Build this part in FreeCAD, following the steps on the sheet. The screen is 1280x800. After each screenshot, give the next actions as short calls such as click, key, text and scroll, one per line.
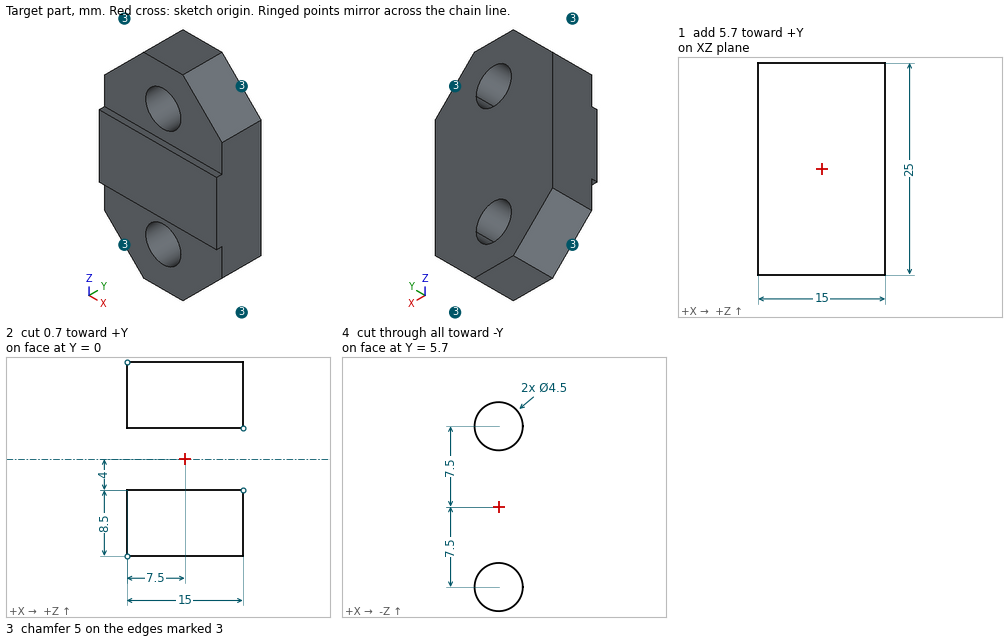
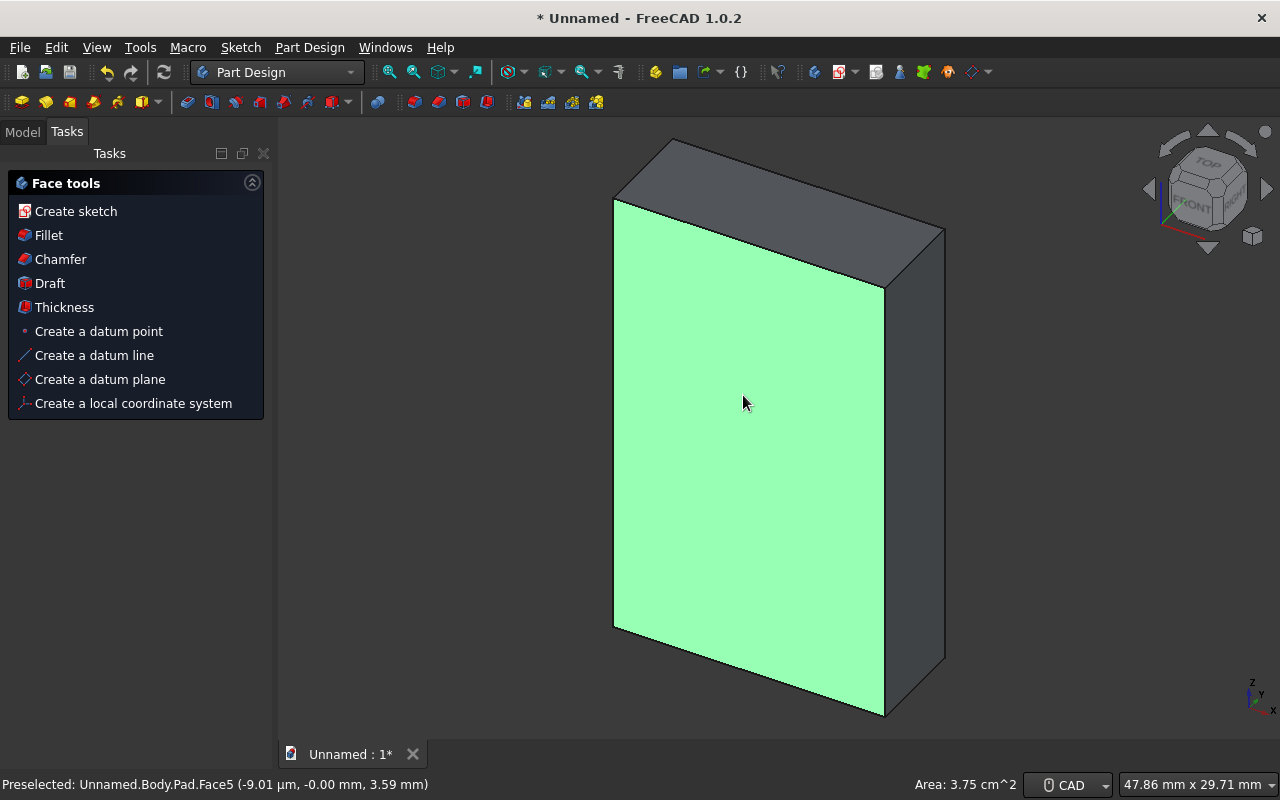
click(840, 72)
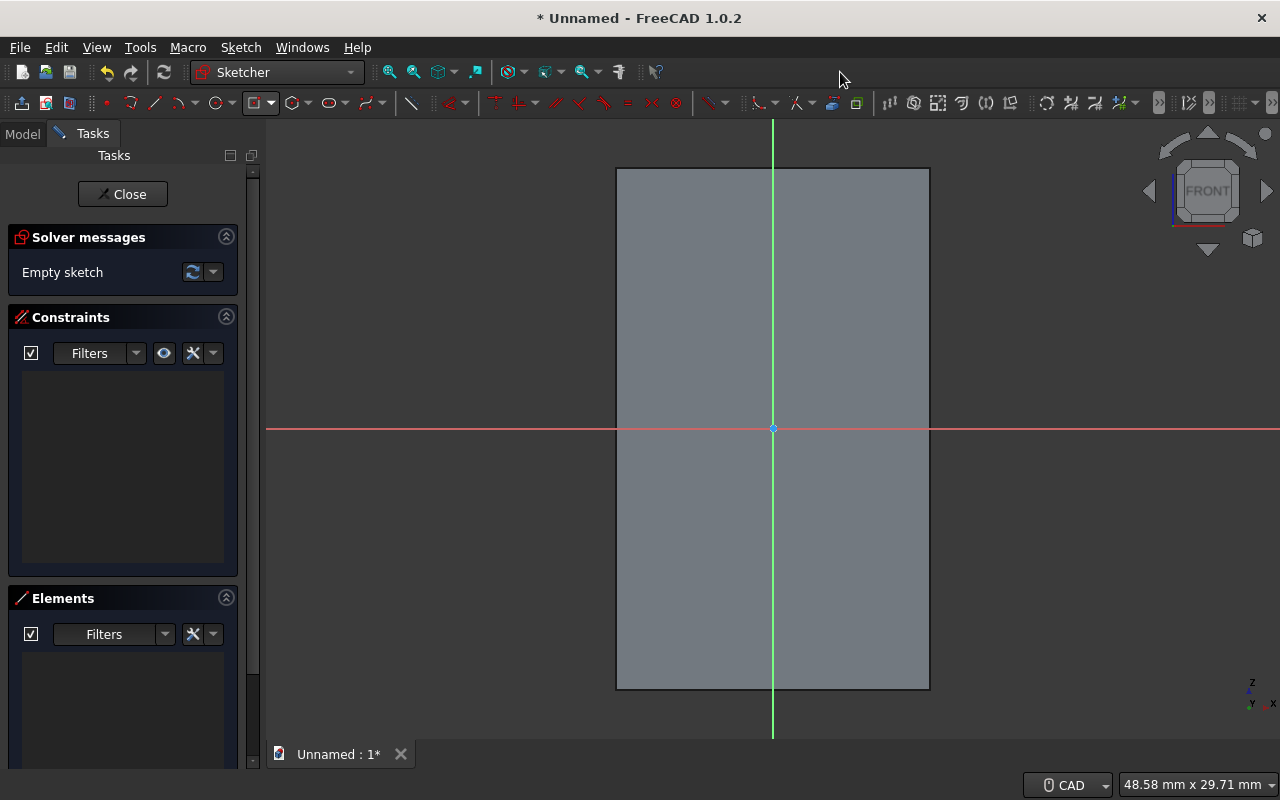
scroll(395, 429, down, 1)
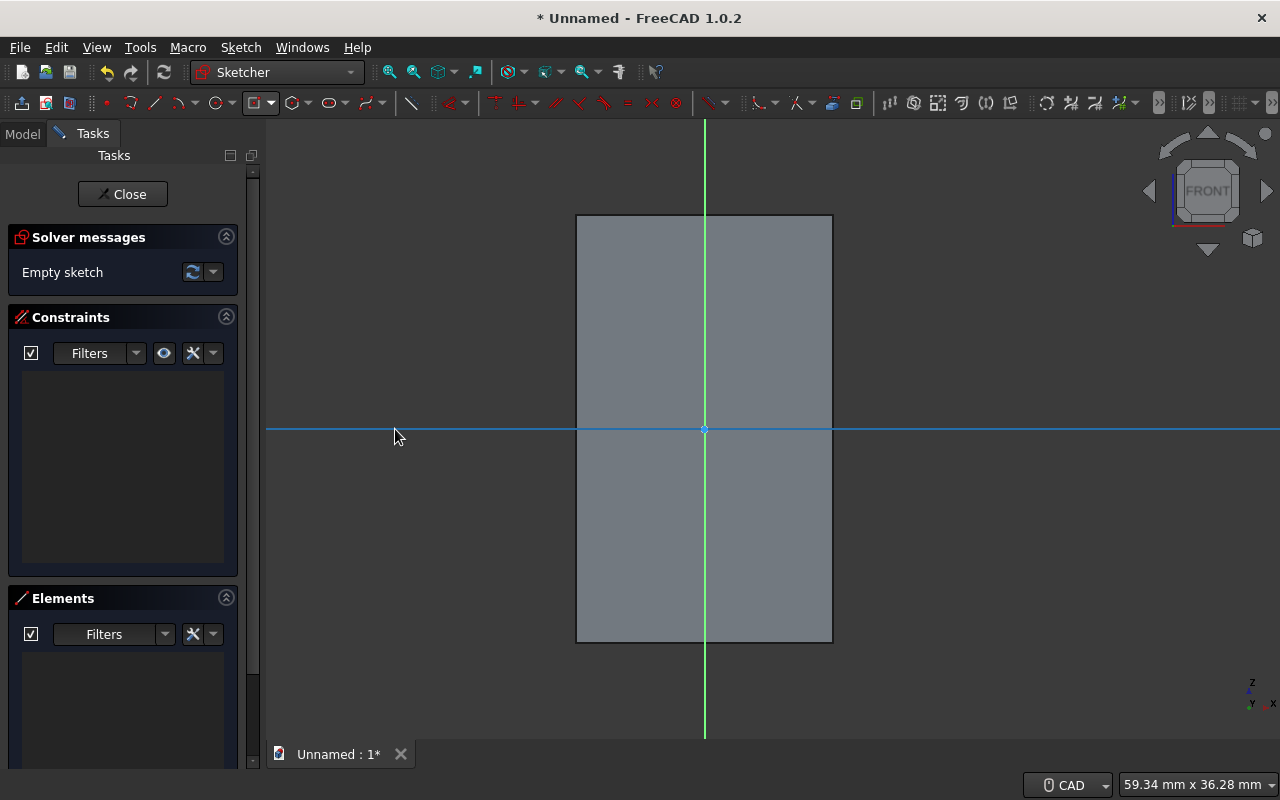
key(g)
key(r)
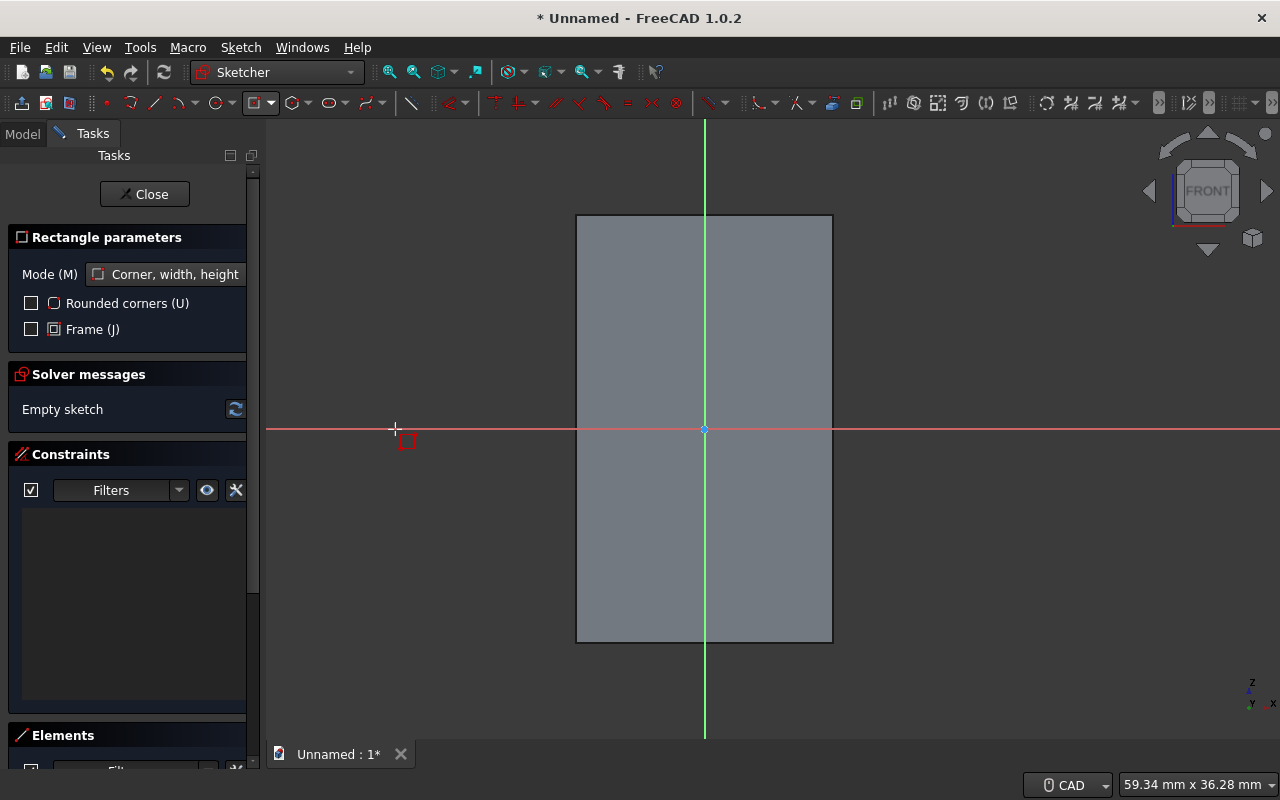
click(576, 497)
click(833, 643)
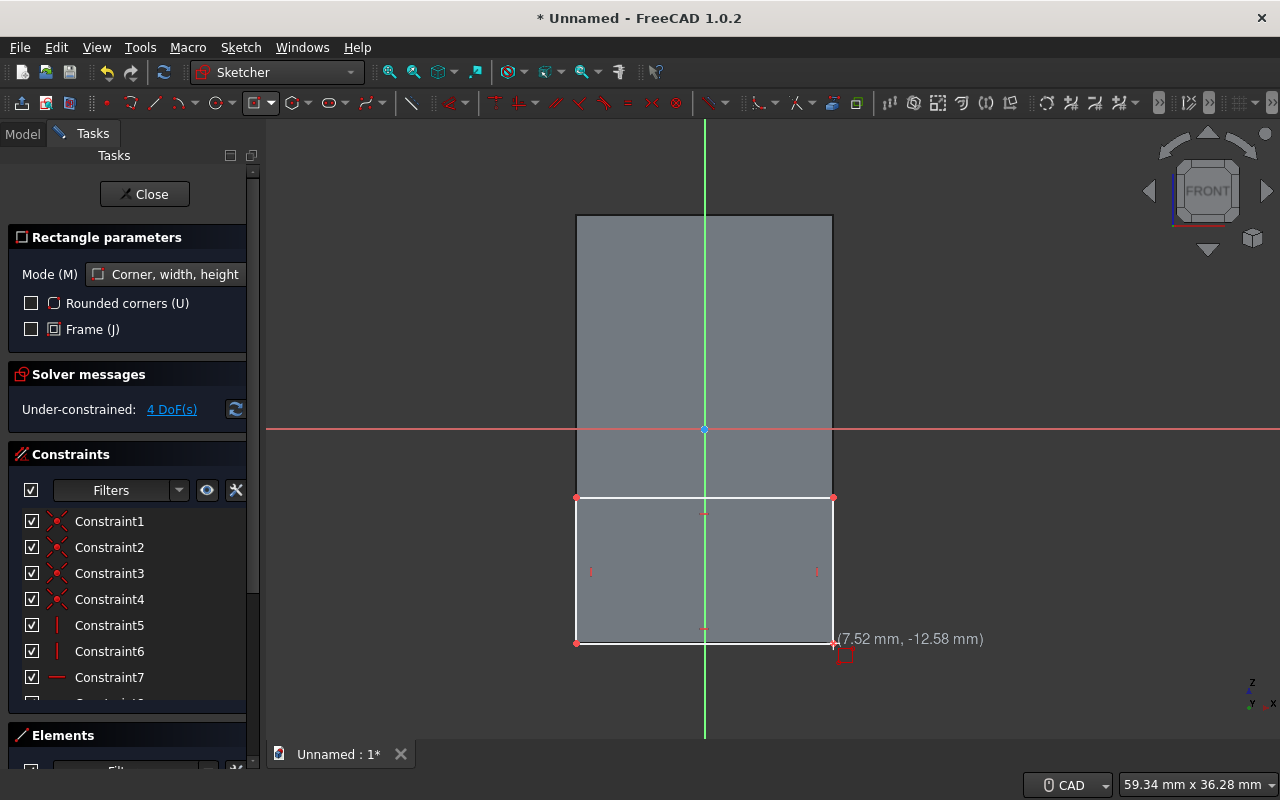
click(576, 215)
click(833, 361)
key(Escape)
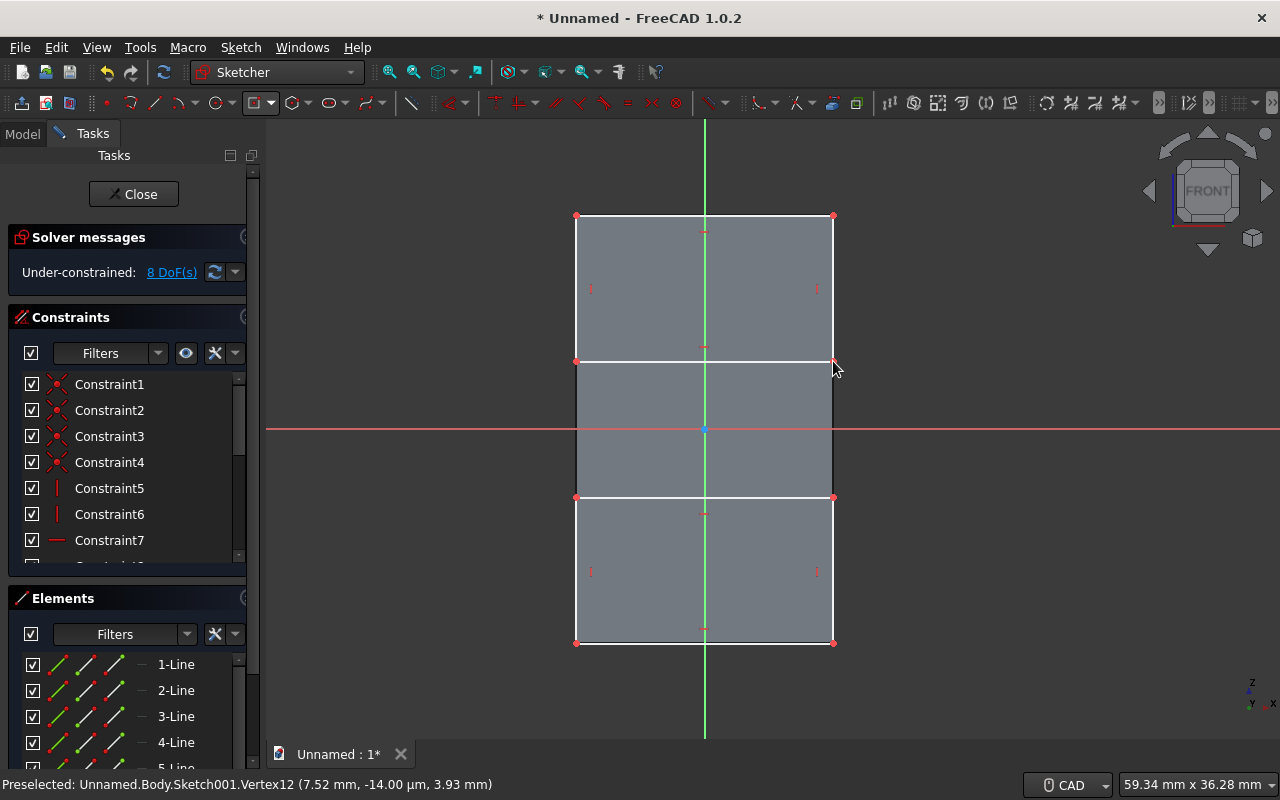
click(576, 644)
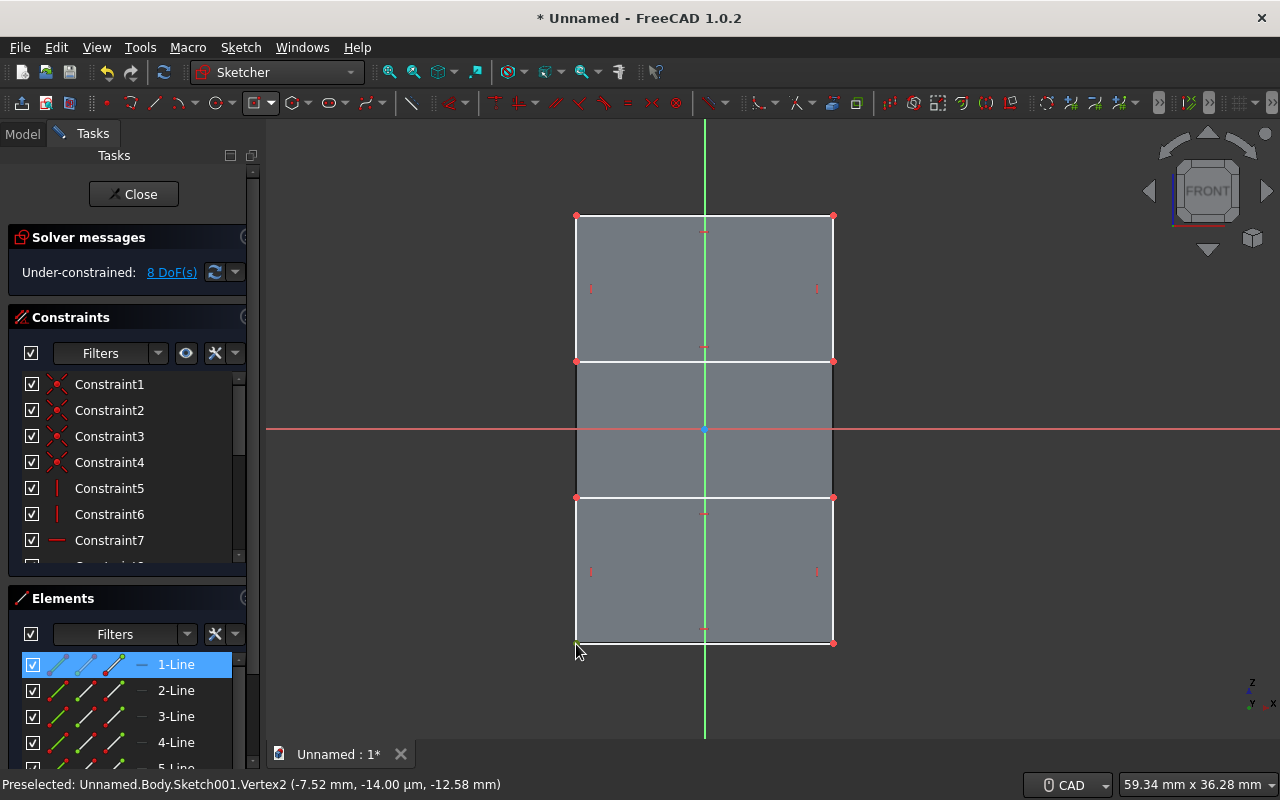
click(576, 216)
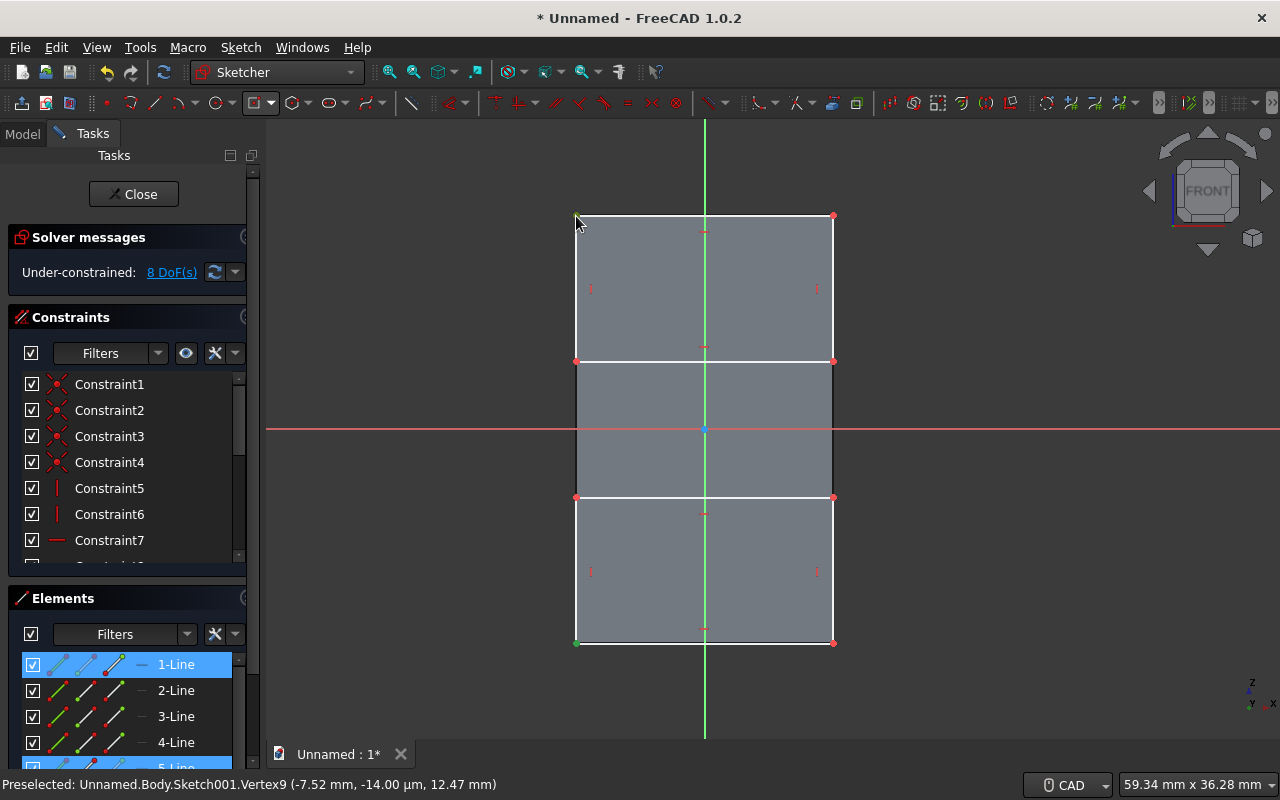
click(353, 429)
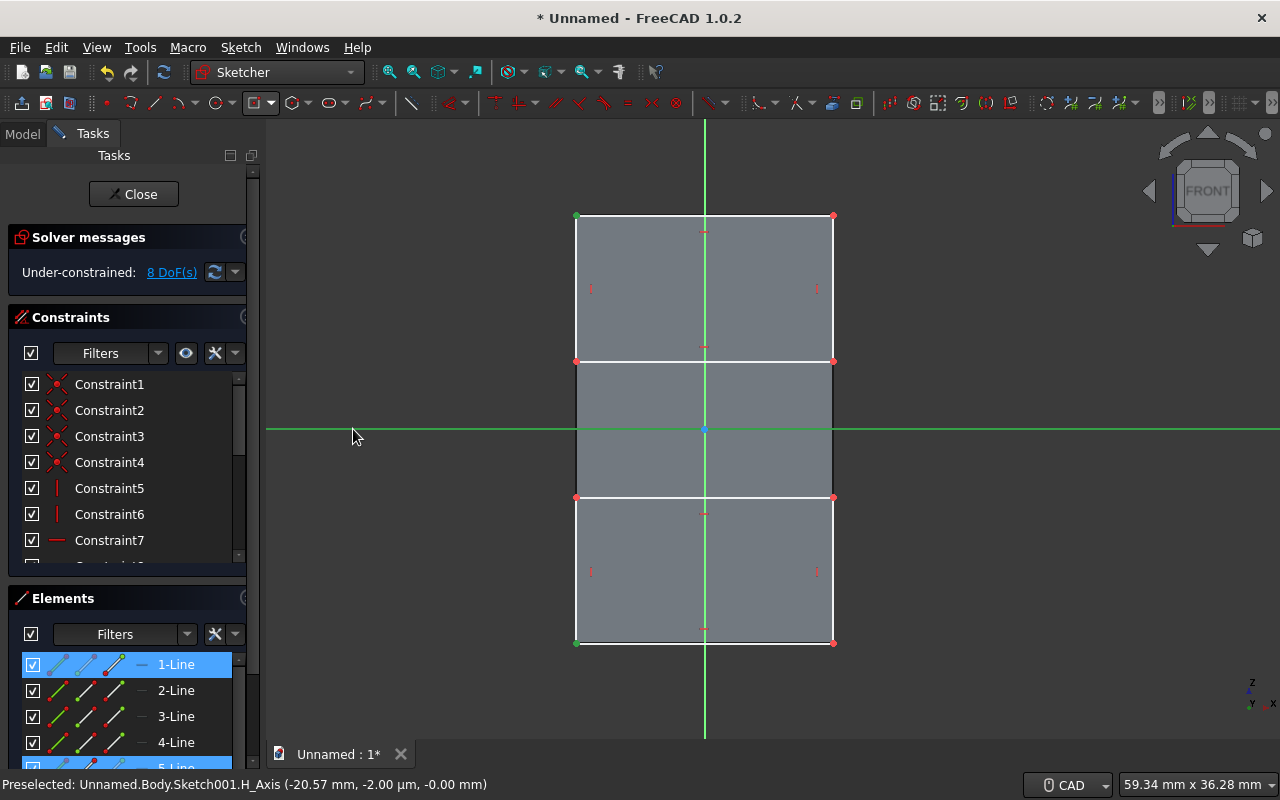
click(652, 104)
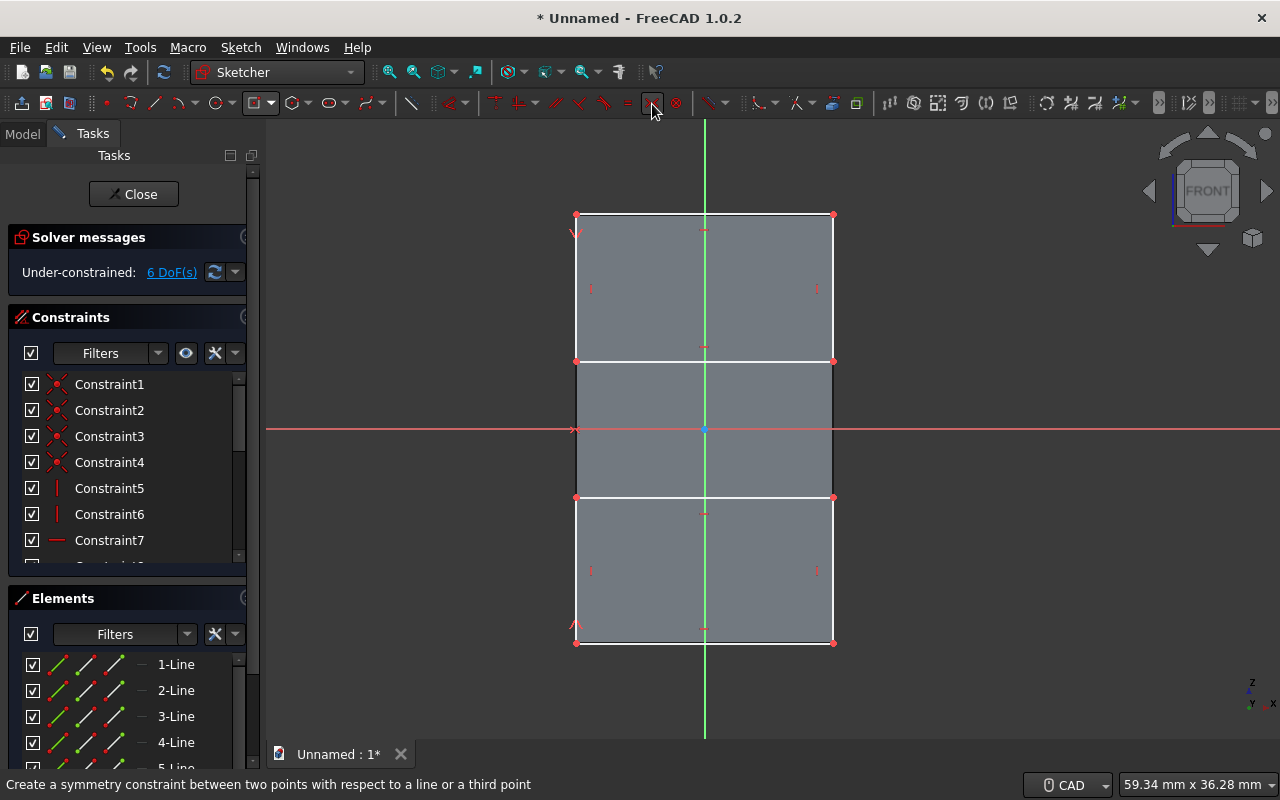
click(833, 498)